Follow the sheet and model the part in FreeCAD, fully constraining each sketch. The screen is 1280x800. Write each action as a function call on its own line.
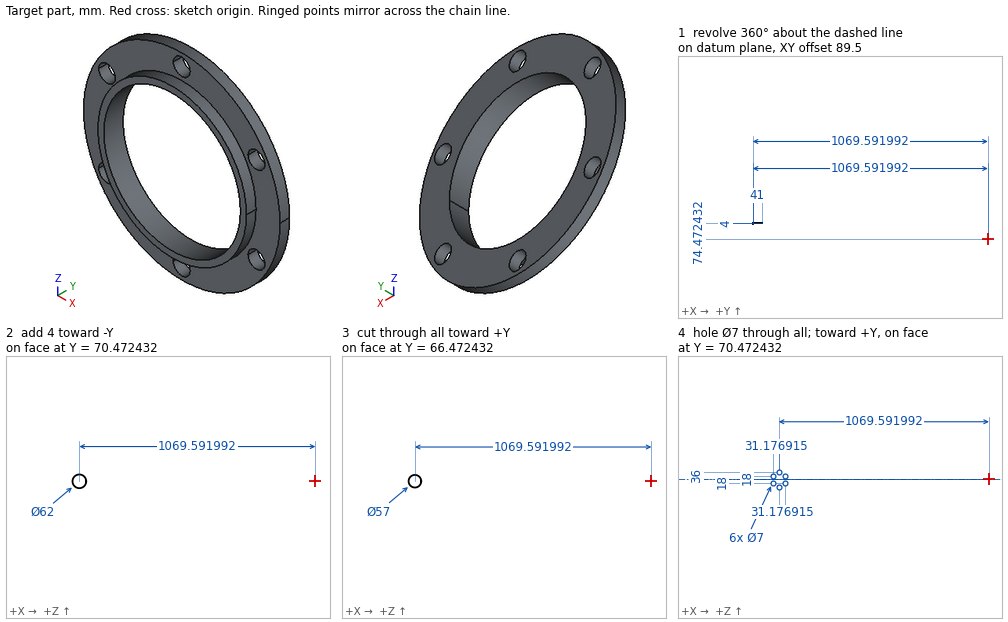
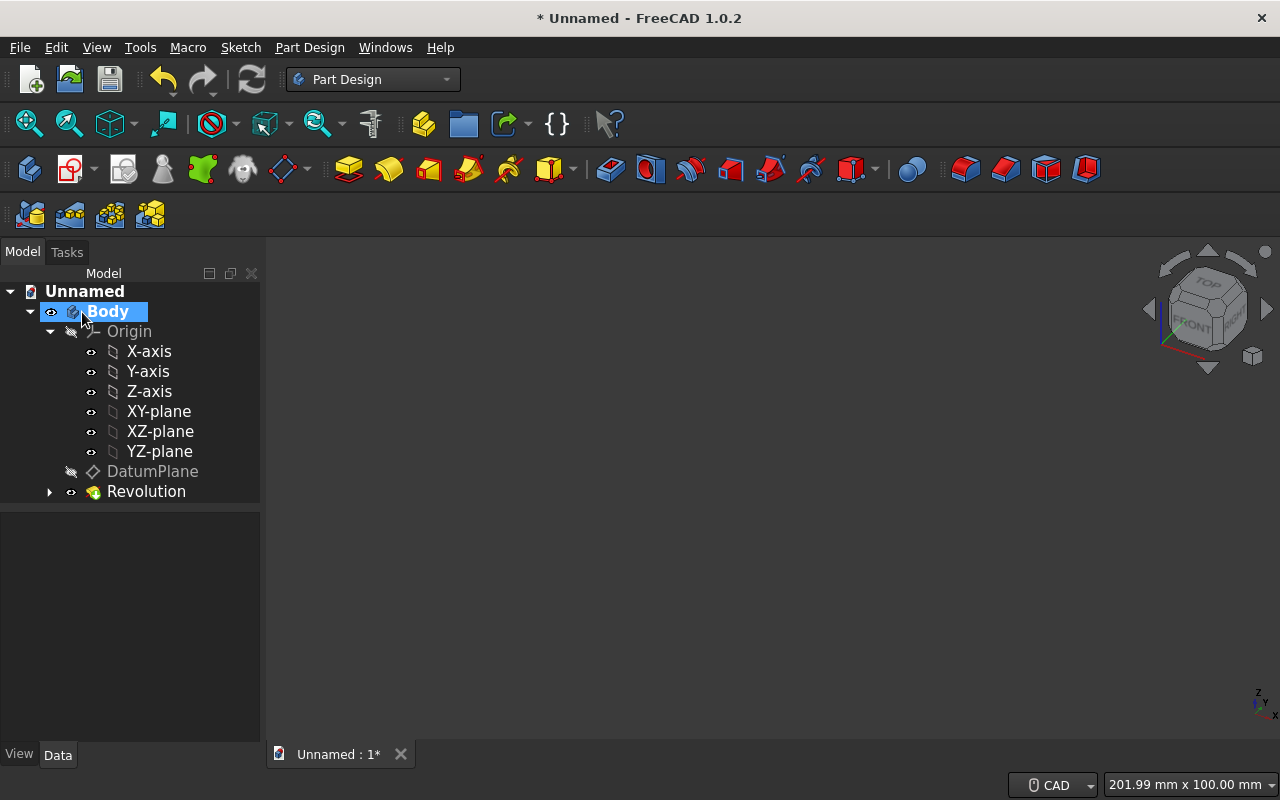
click(30, 124)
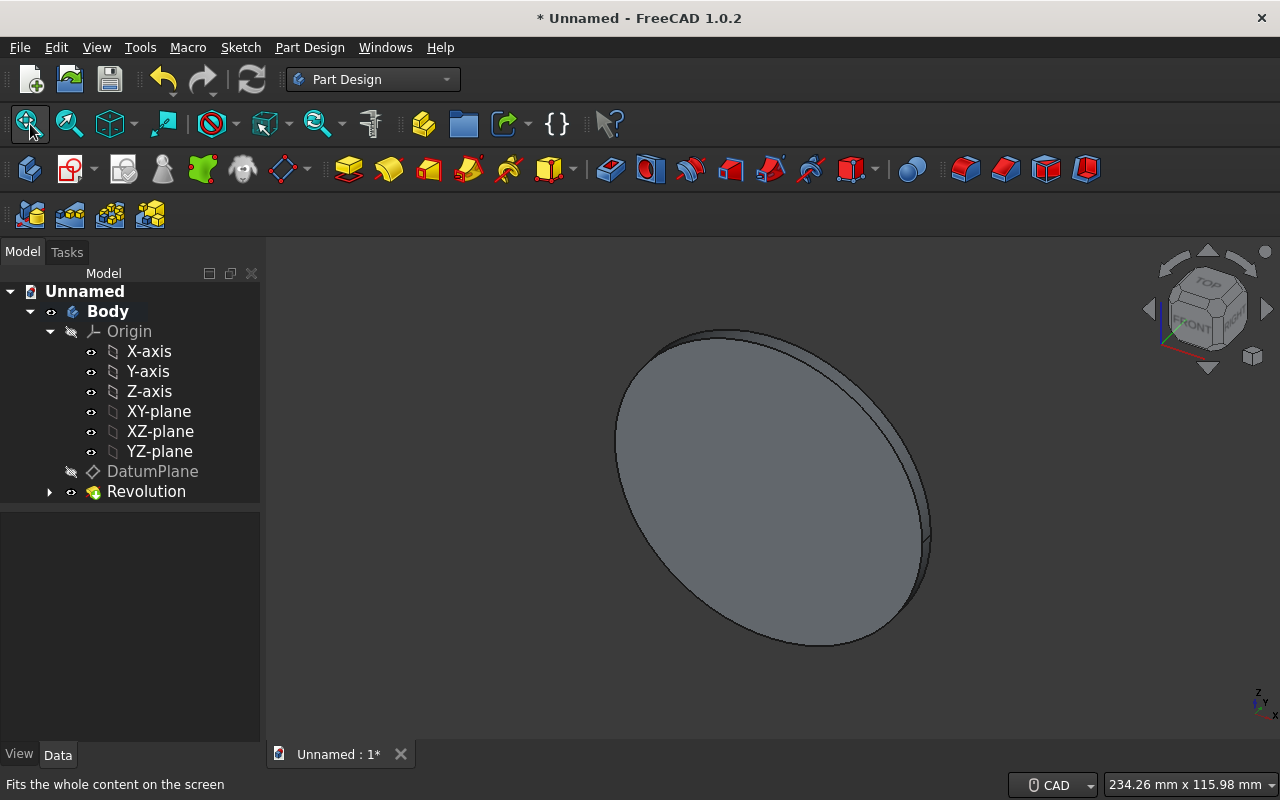
click(769, 491)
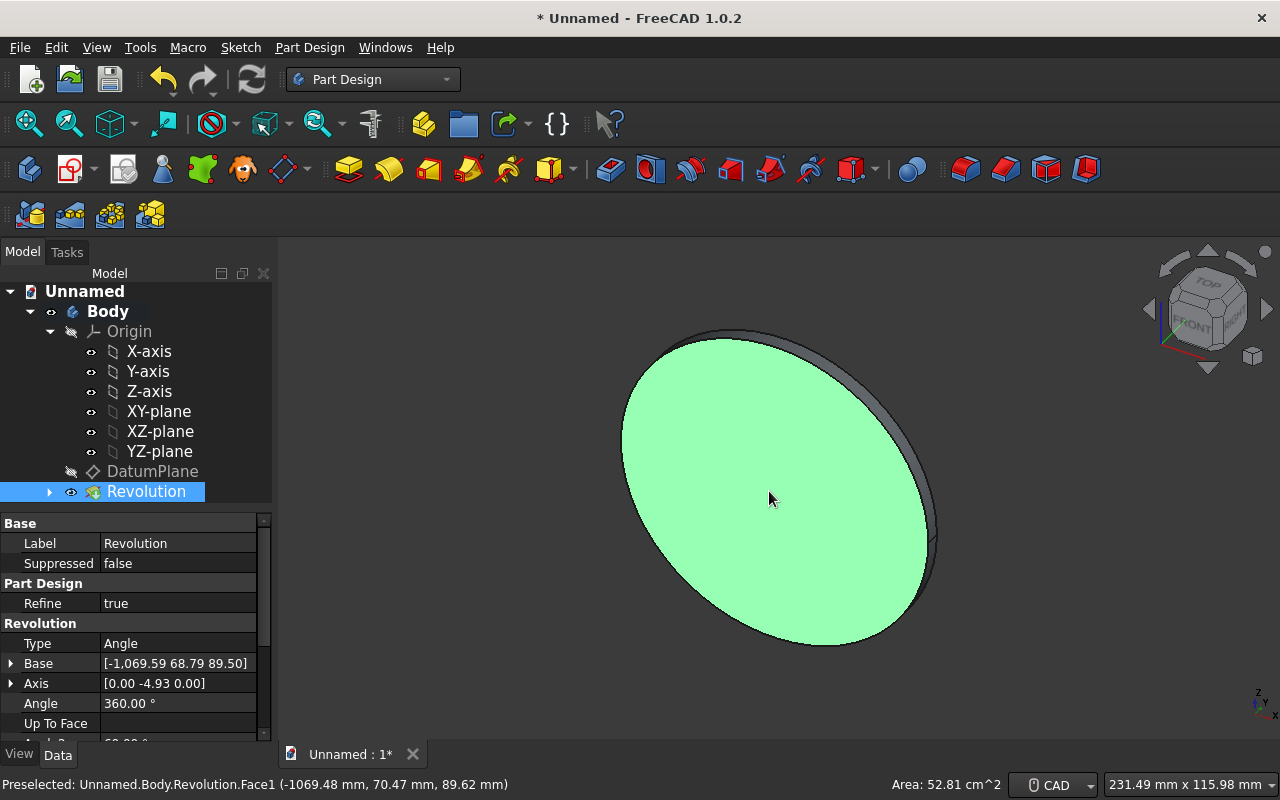
click(70, 170)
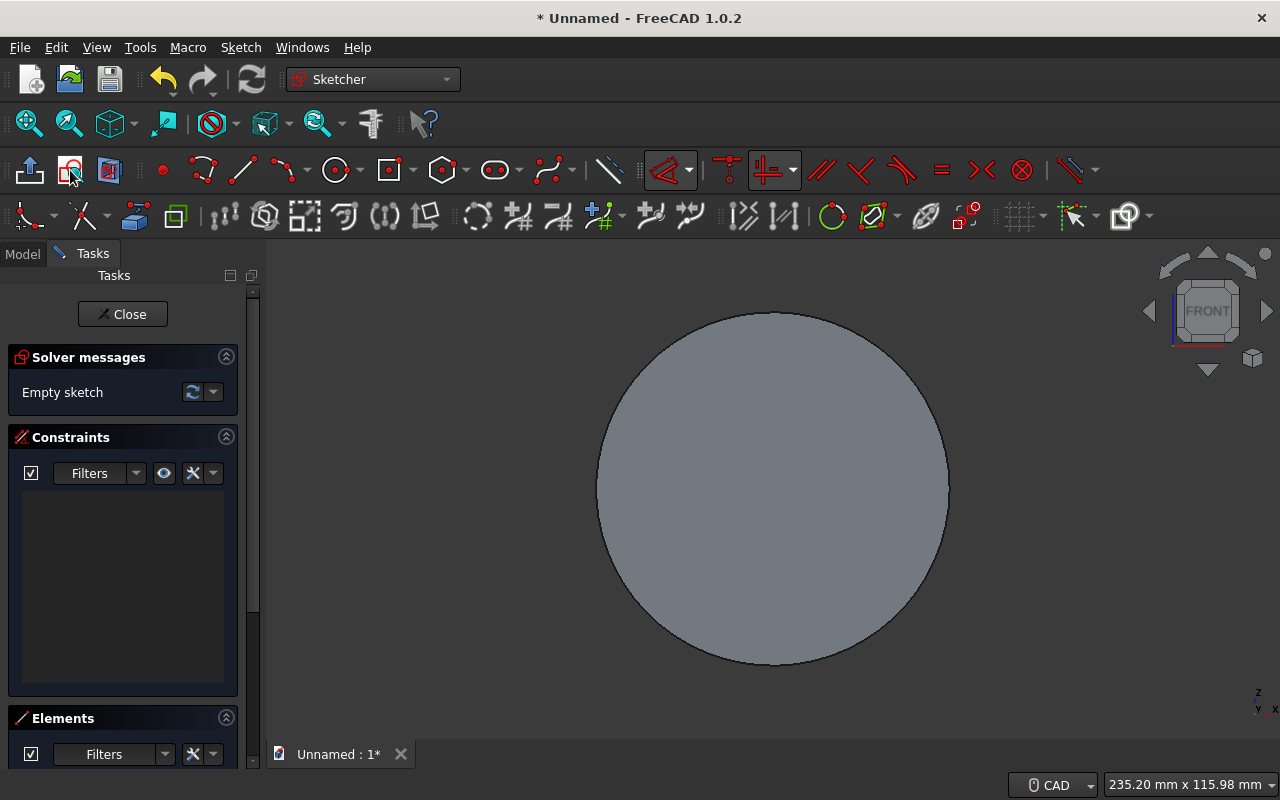
click(336, 170)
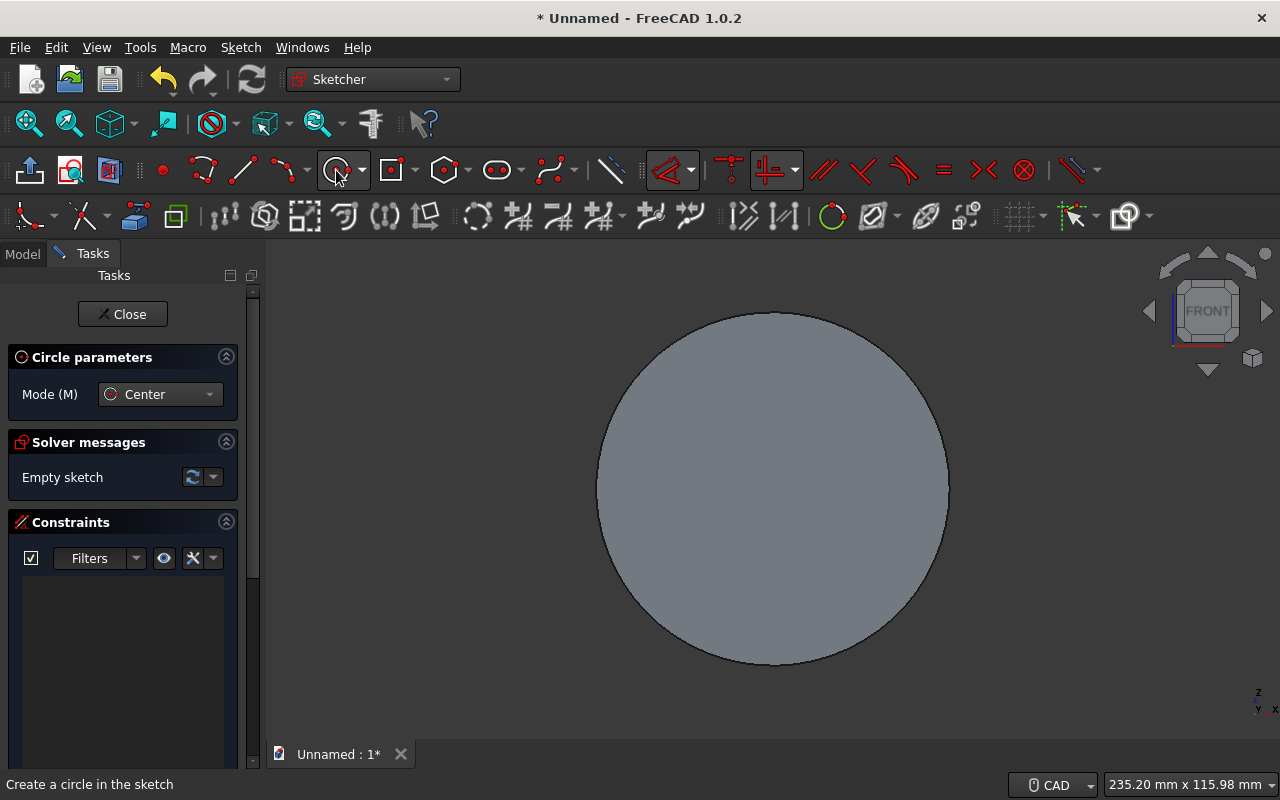
click(773, 489)
move(867, 394)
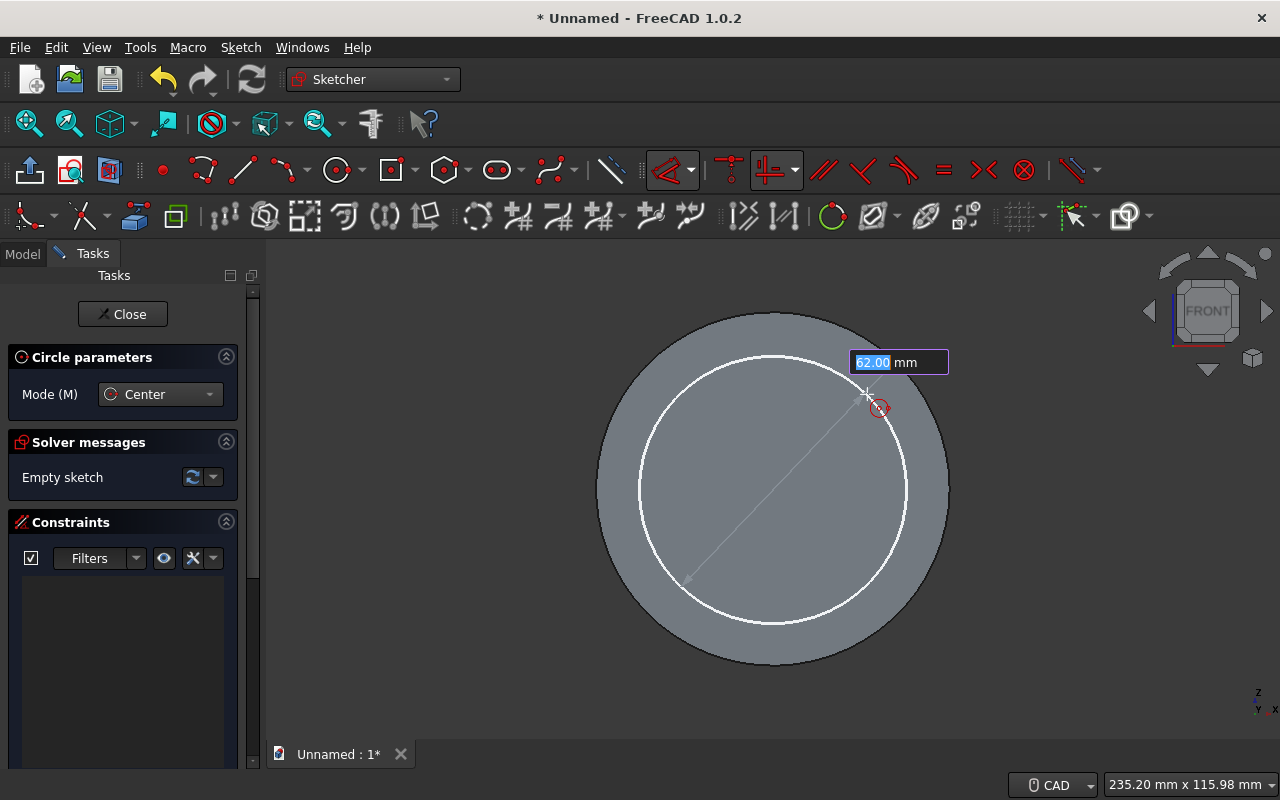
text(62)
key(Return)
key(Escape)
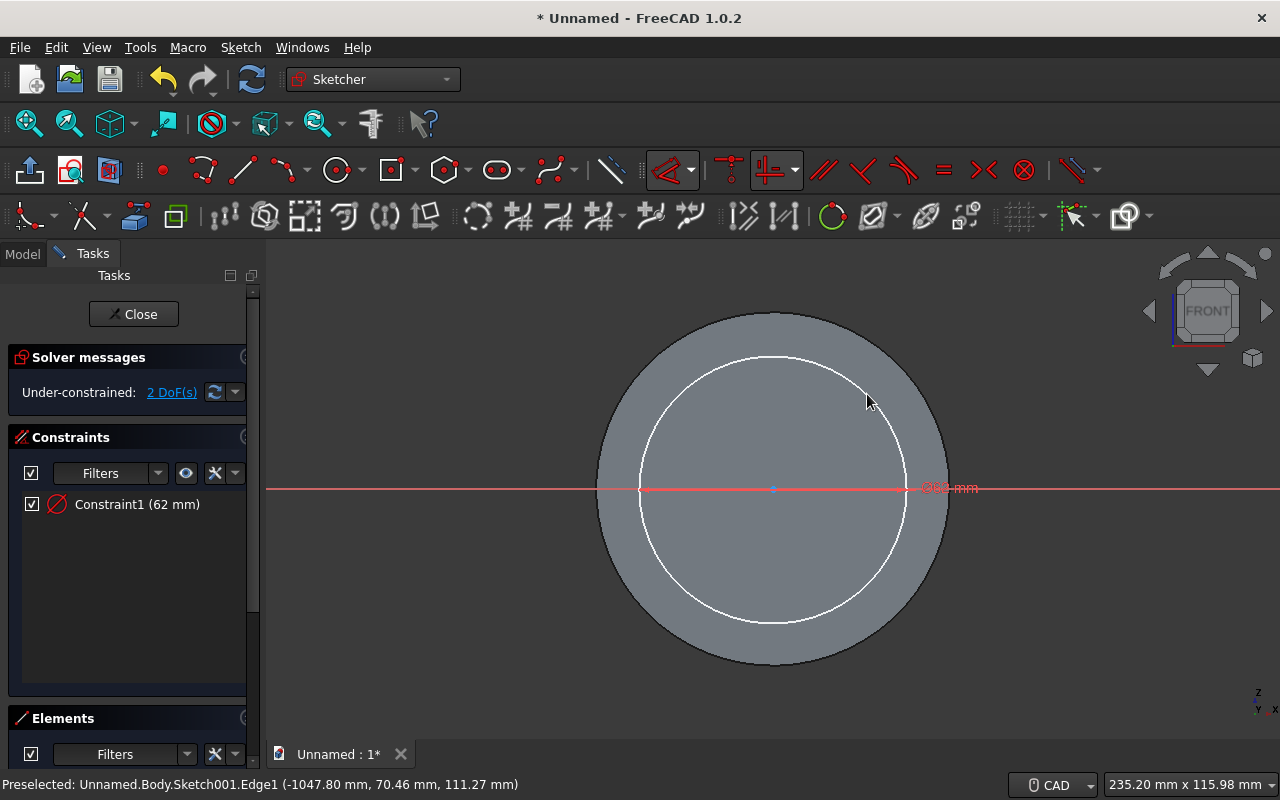
click(773, 490)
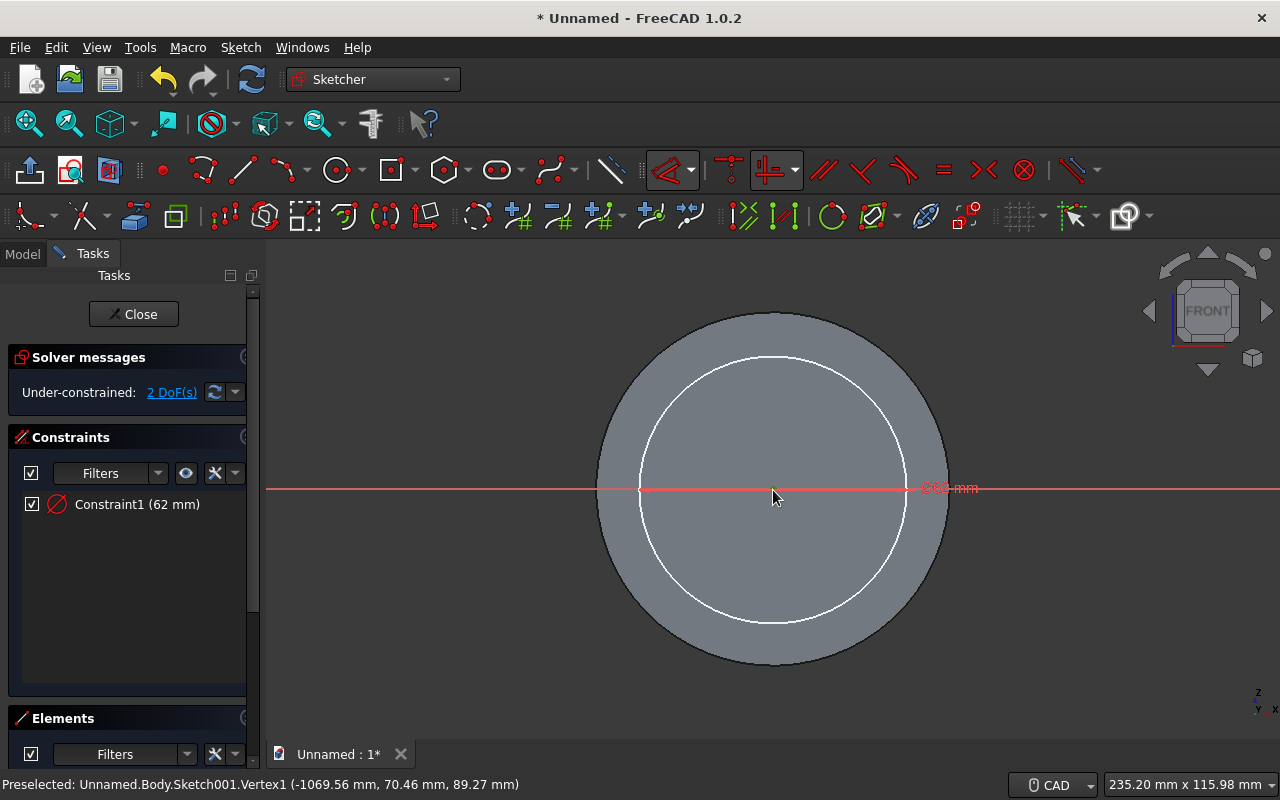
click(353, 489)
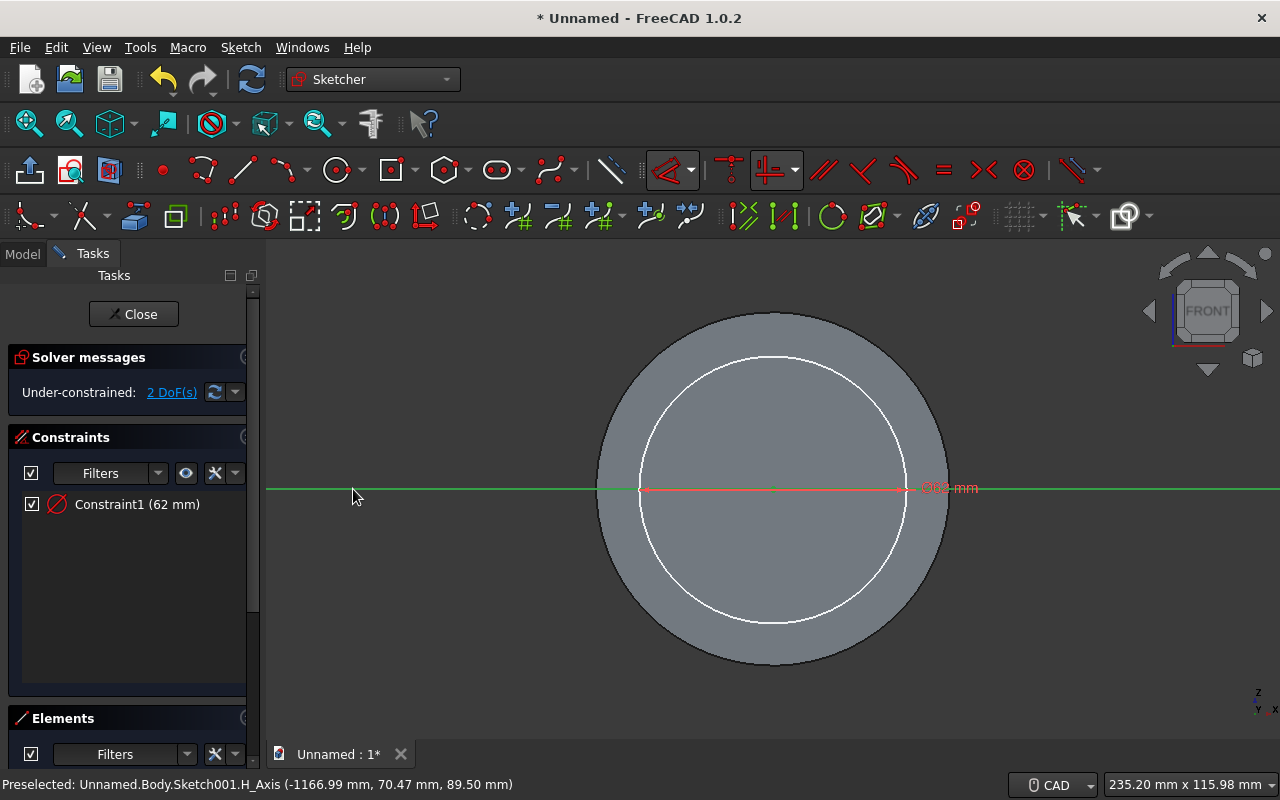
click(730, 170)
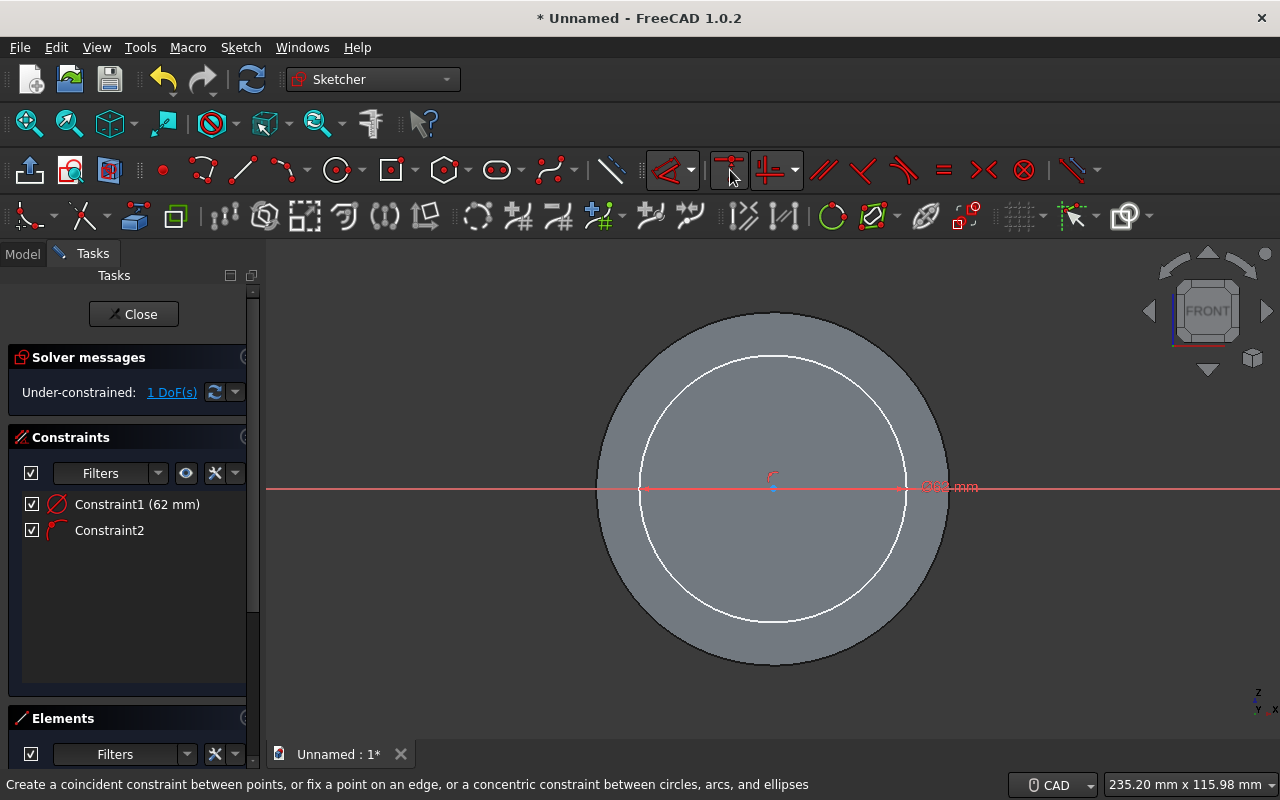
click(773, 489)